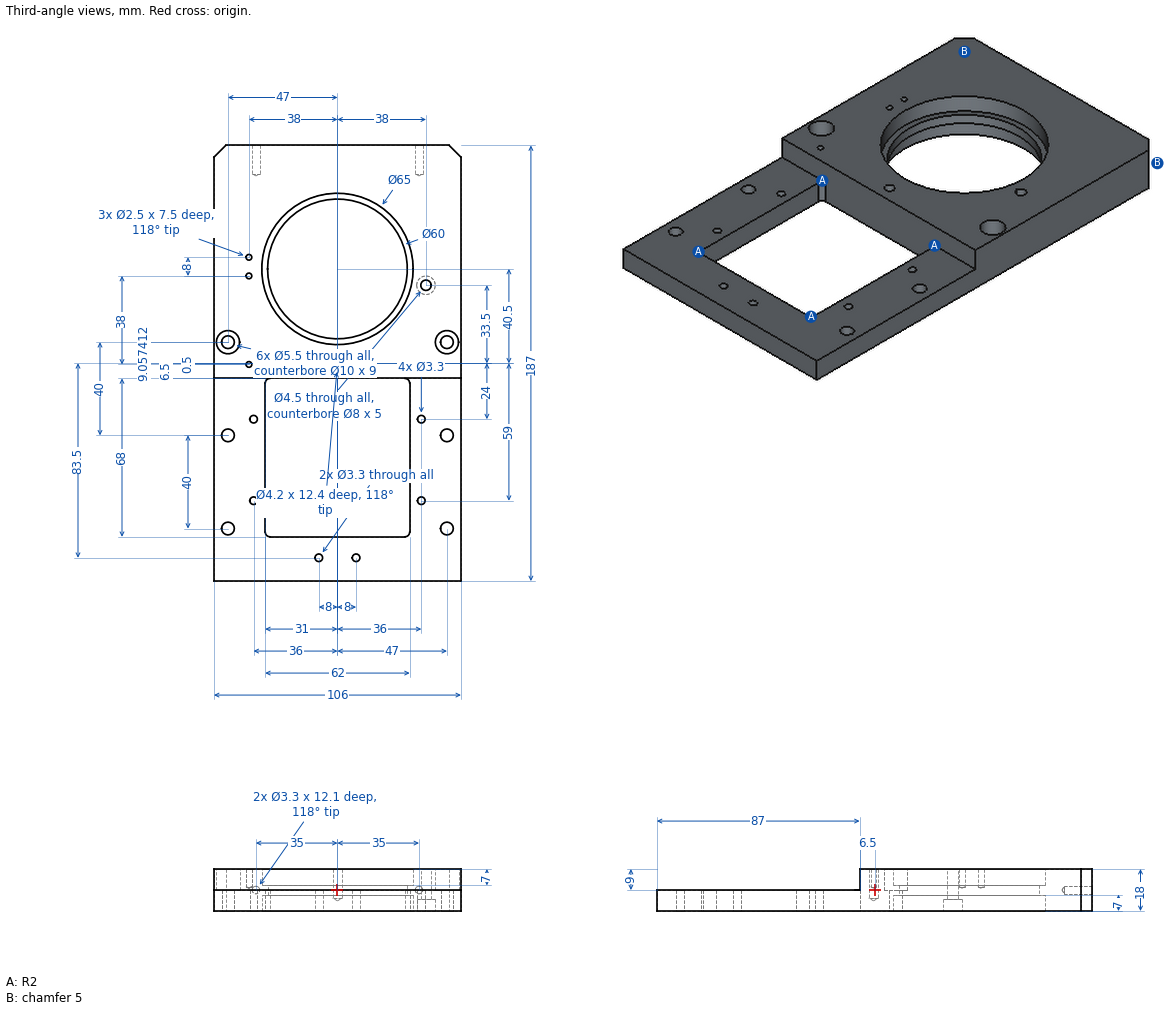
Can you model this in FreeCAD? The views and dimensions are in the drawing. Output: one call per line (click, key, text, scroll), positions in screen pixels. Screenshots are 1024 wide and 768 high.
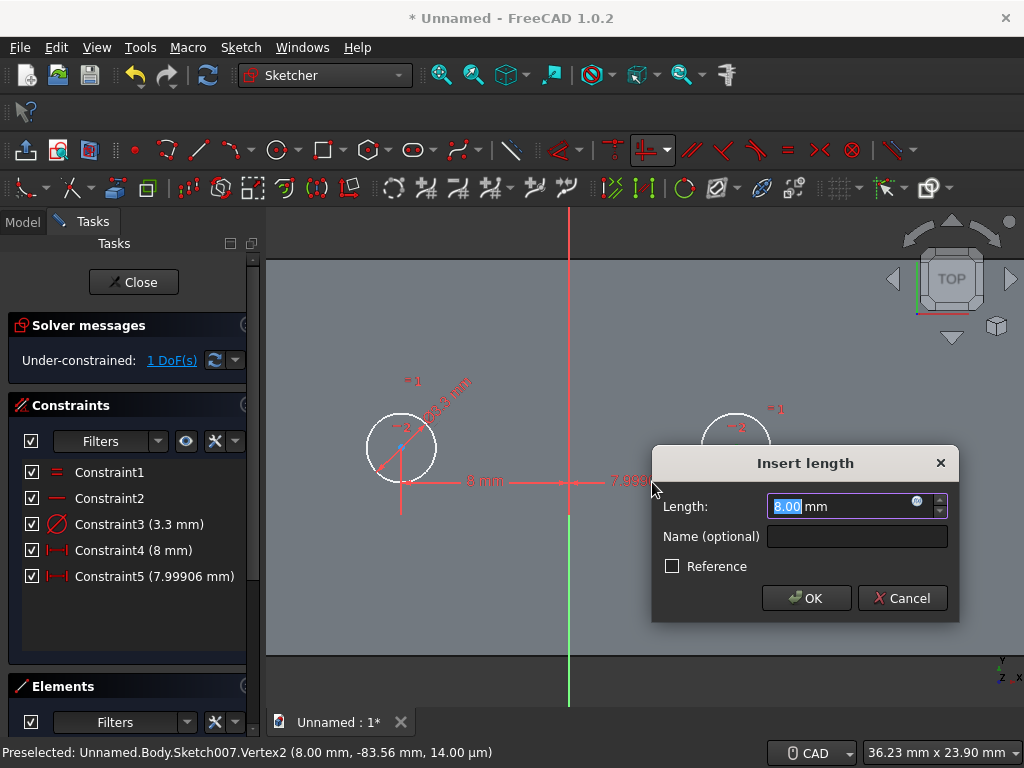
text(8)
key(Return)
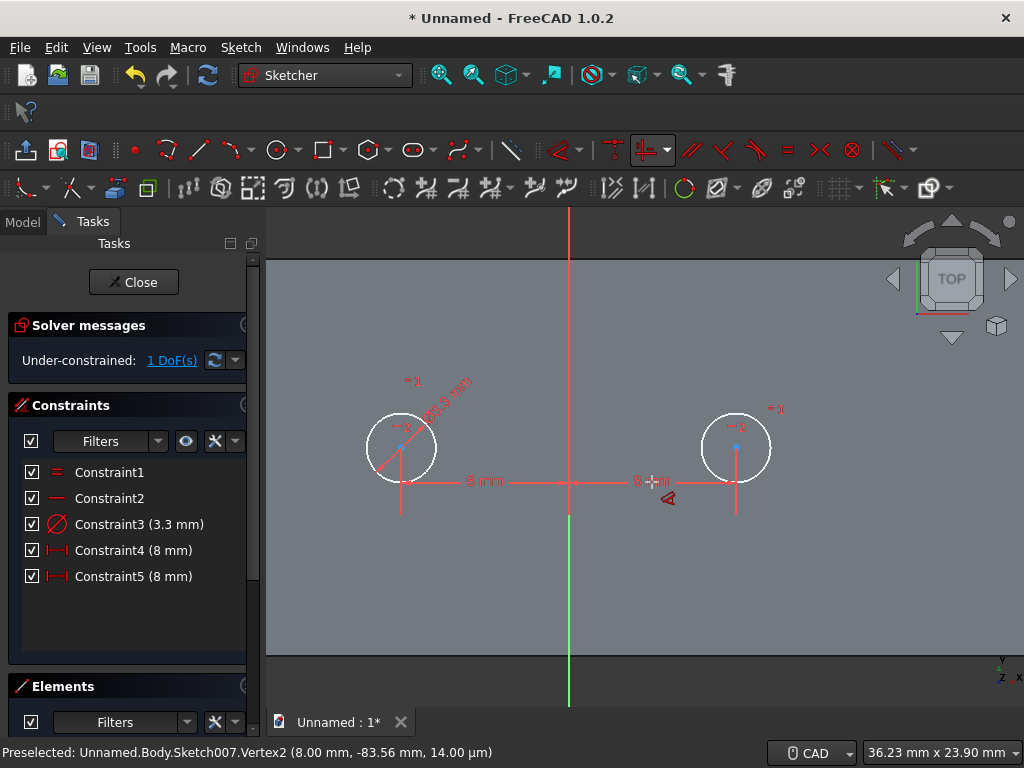
click(401, 448)
click(367, 342)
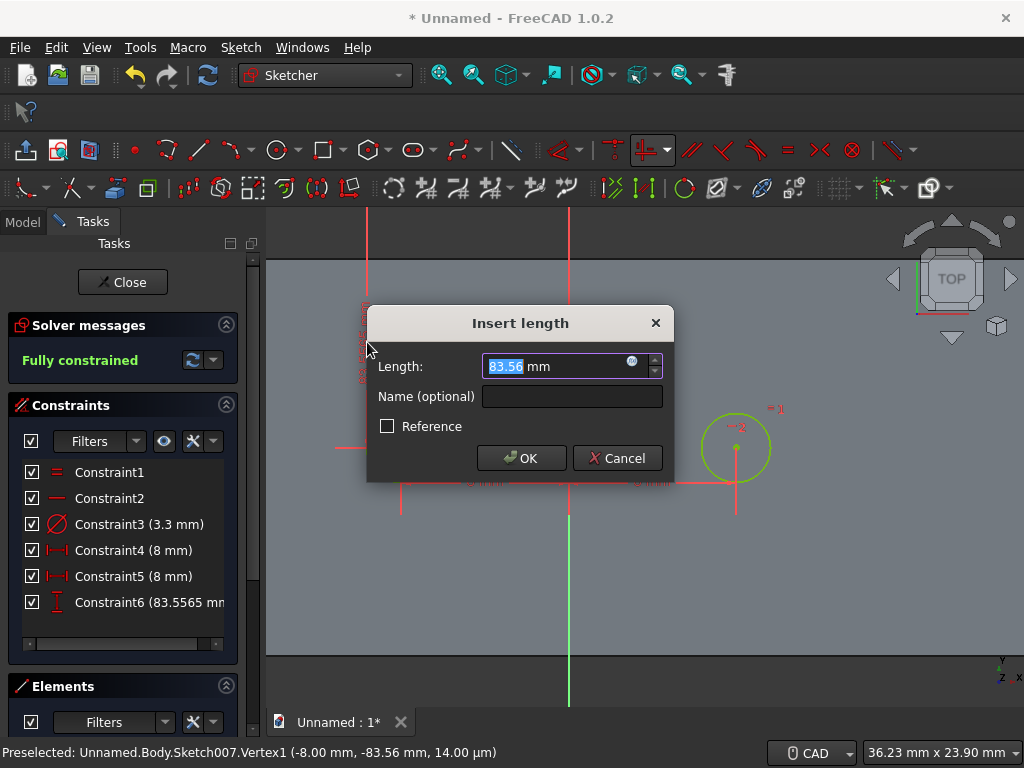
text(83.5)
key(Return)
key(Escape)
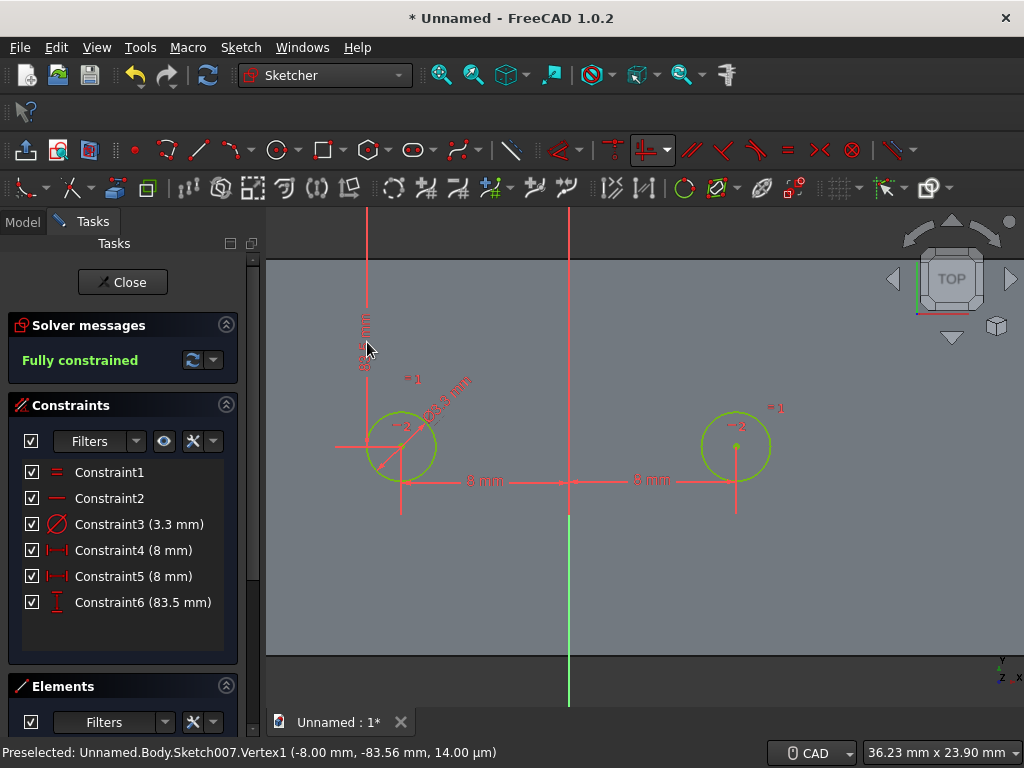
click(123, 282)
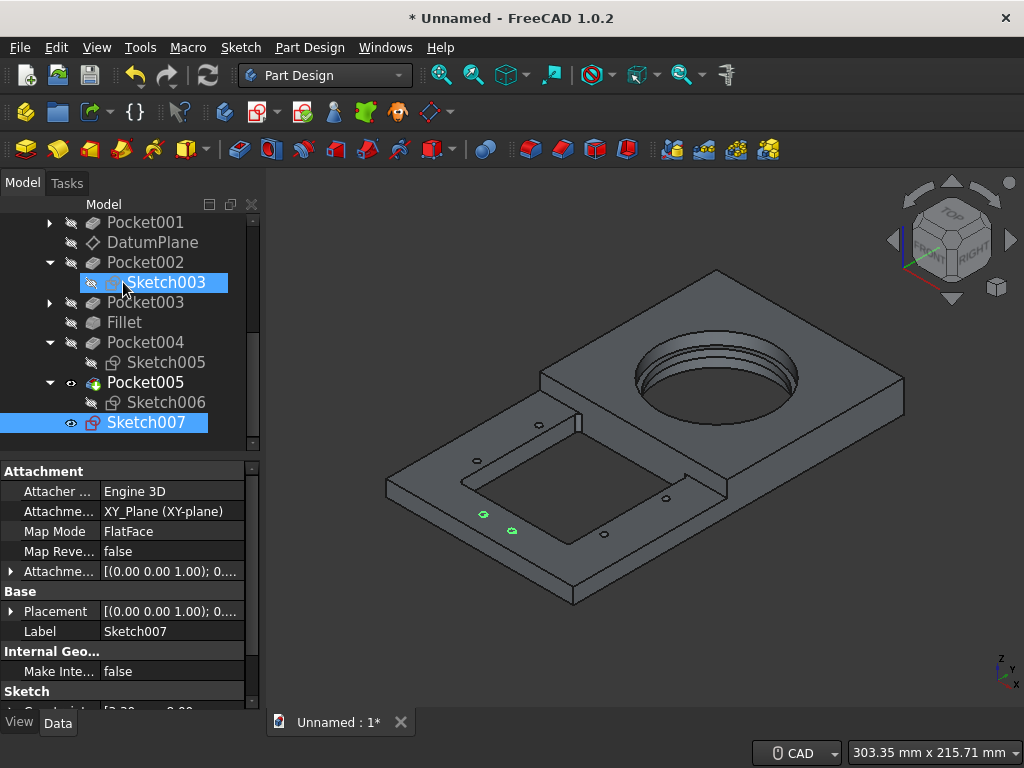
click(272, 150)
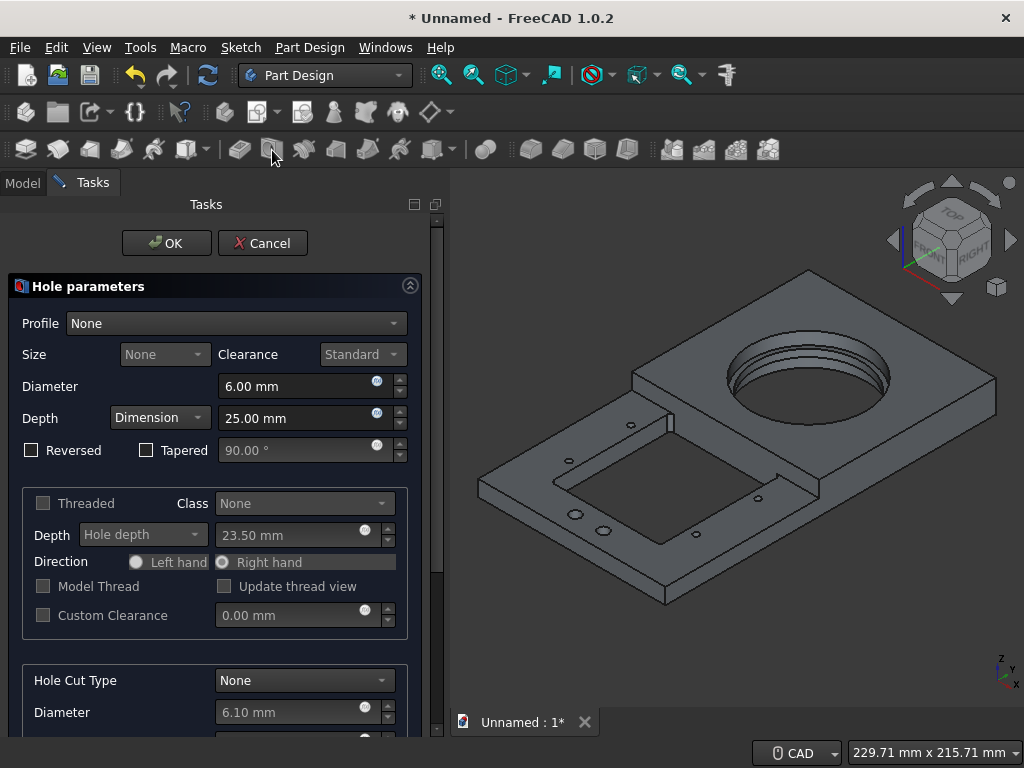
triple_click(305, 386)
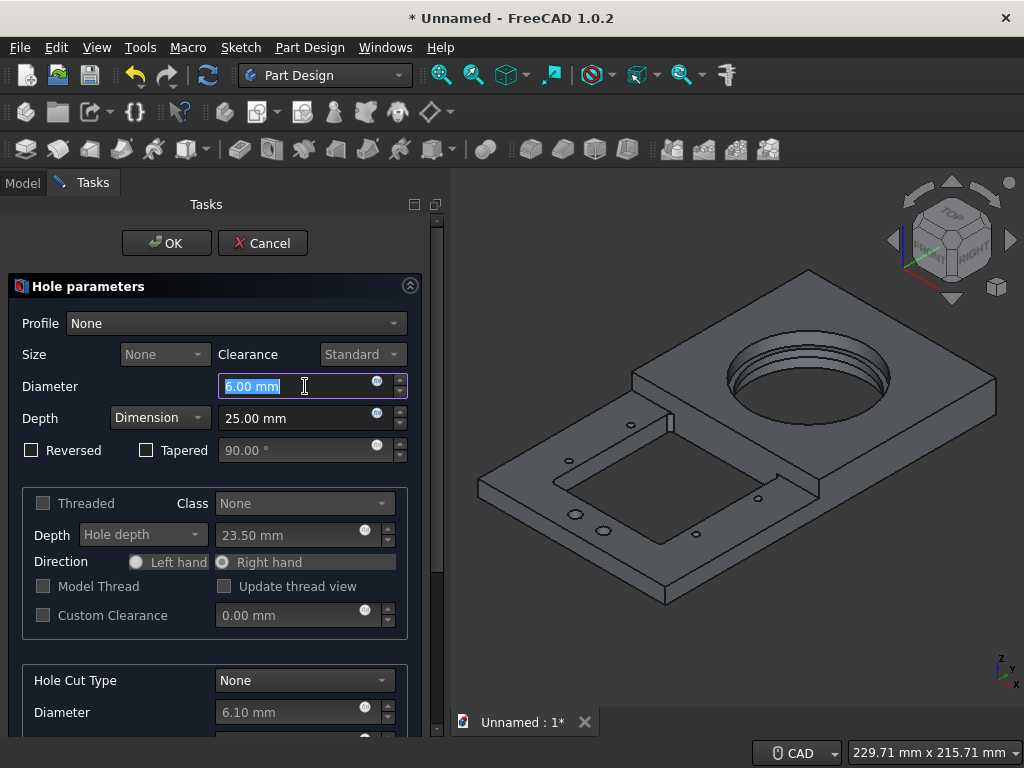
text(3.3)
key(Tab)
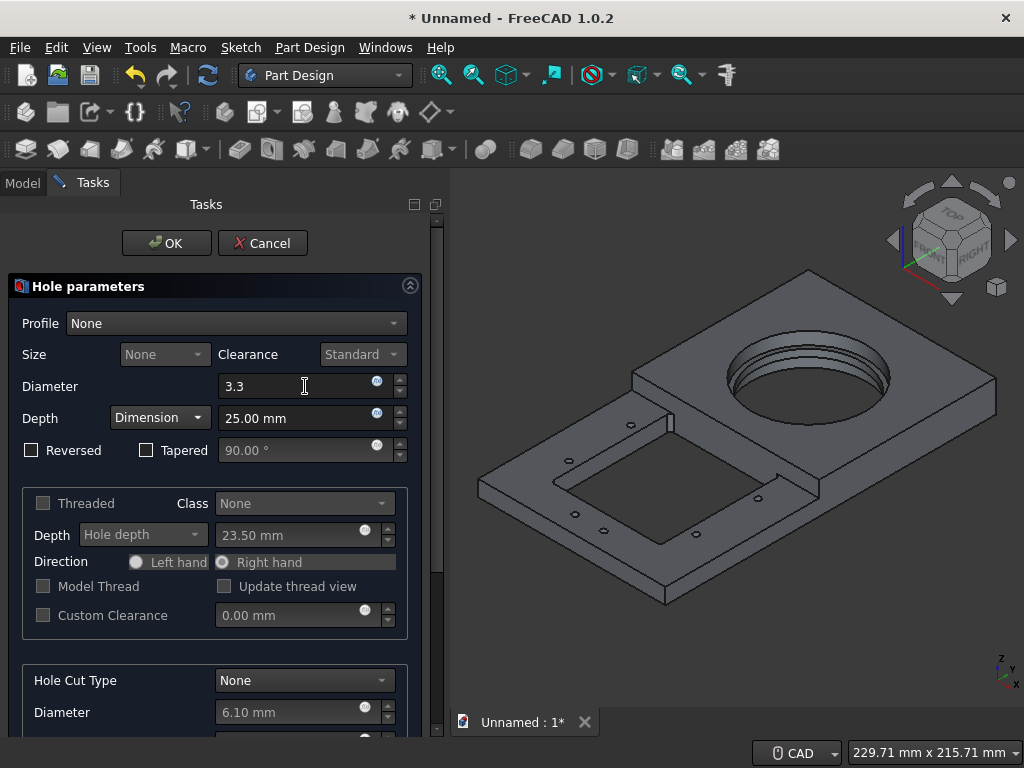
click(161, 418)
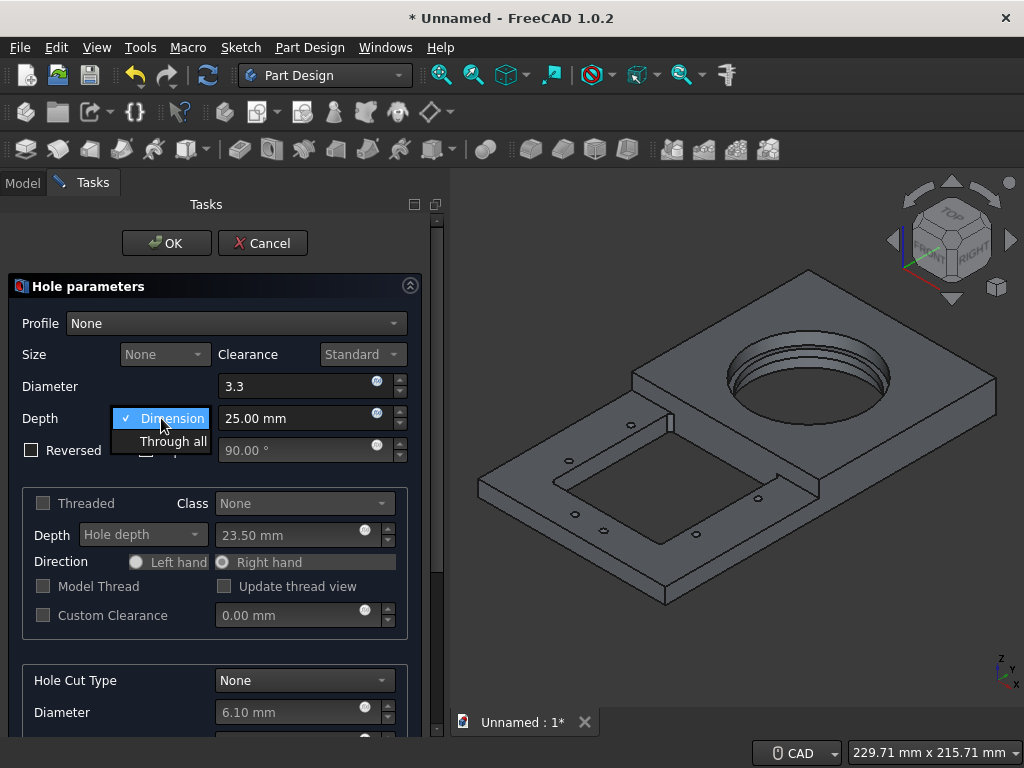
click(160, 442)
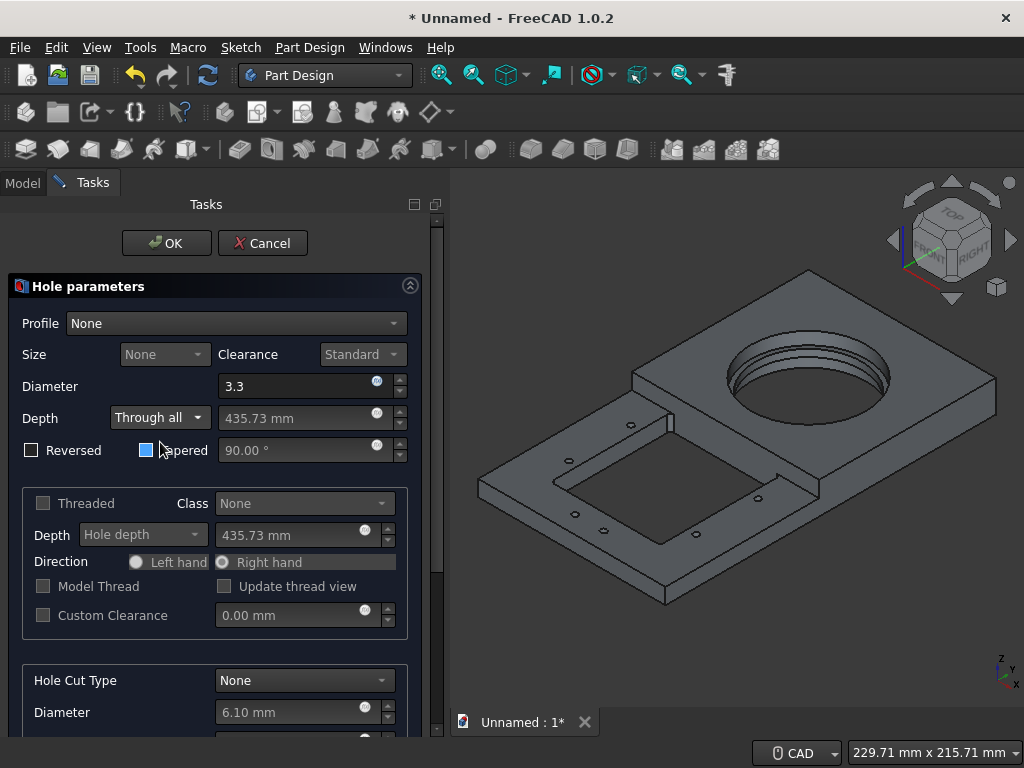
click(167, 243)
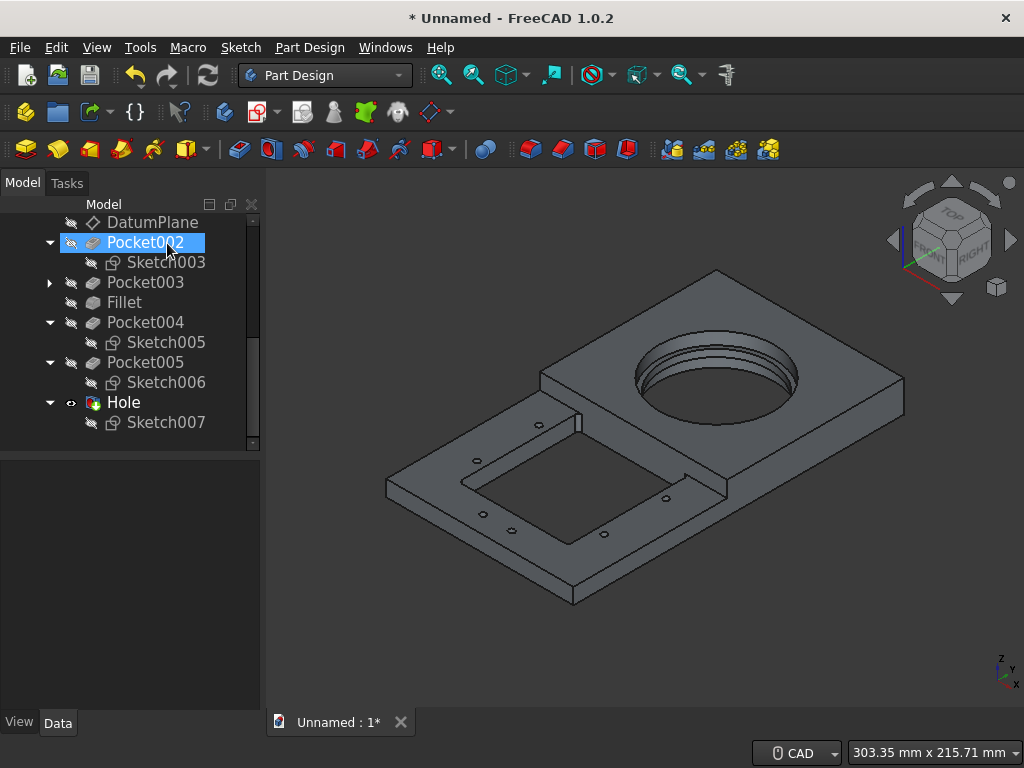
click(826, 376)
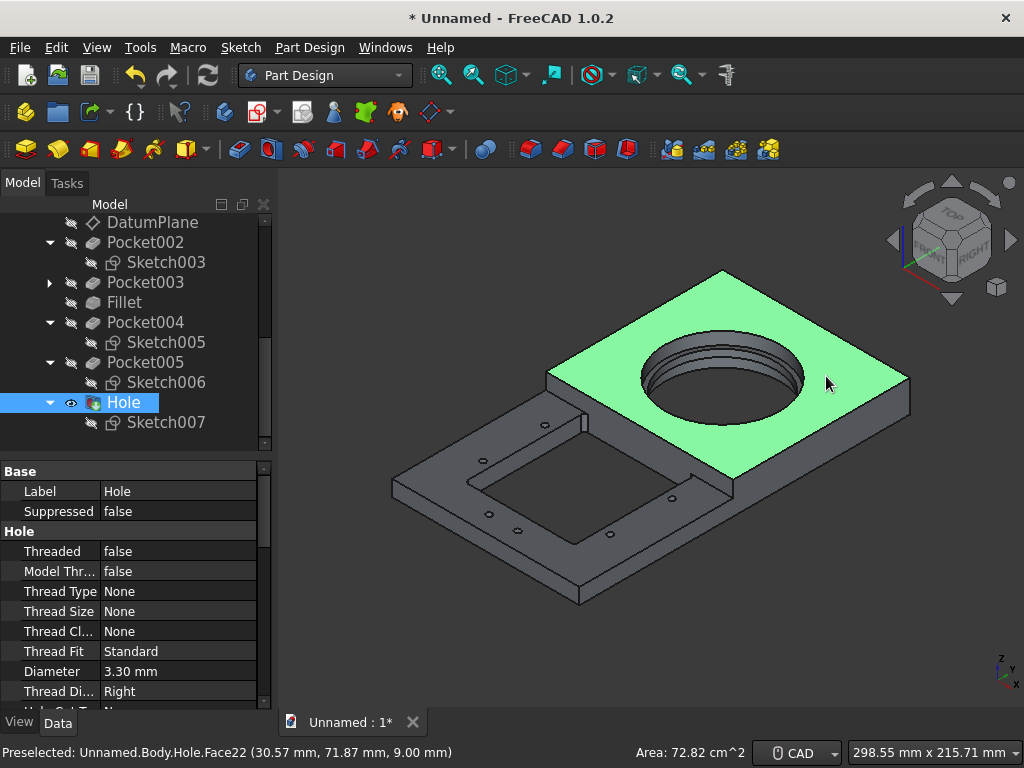
click(258, 112)